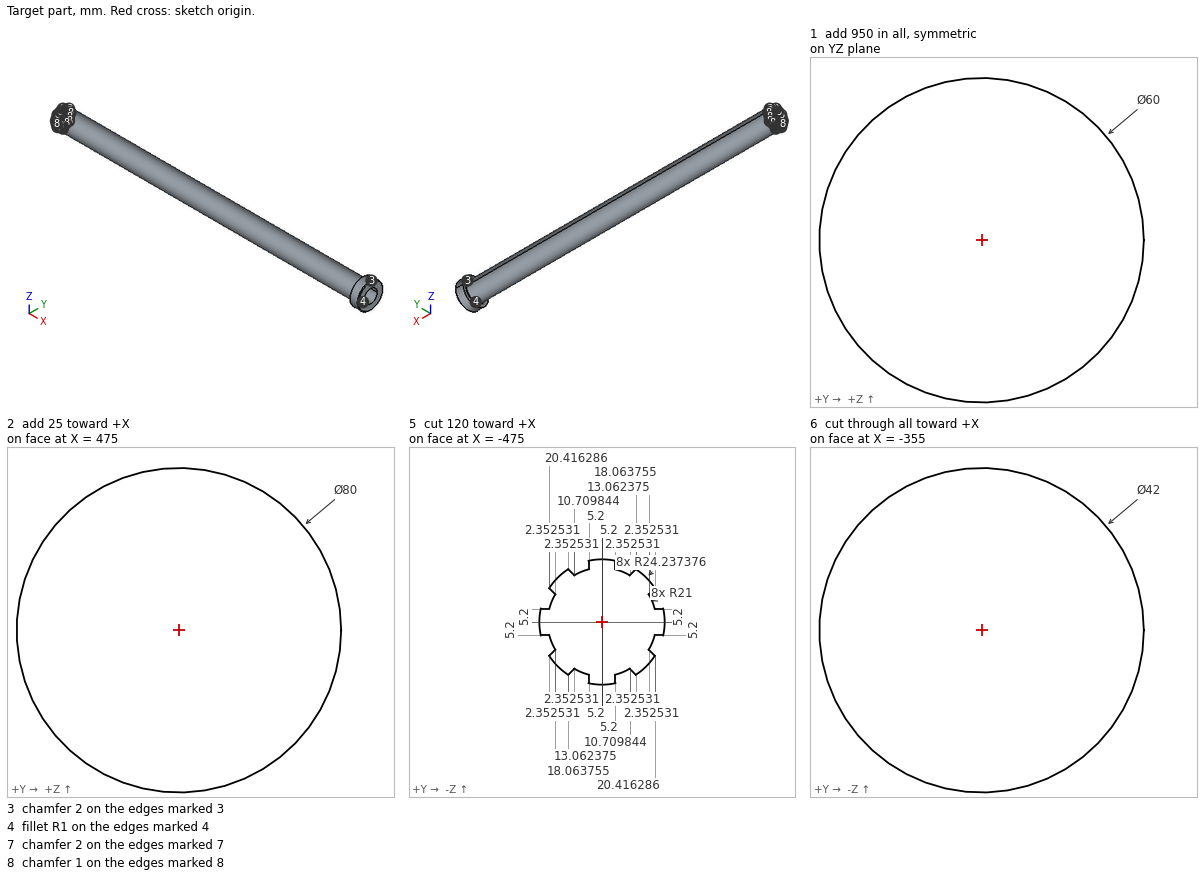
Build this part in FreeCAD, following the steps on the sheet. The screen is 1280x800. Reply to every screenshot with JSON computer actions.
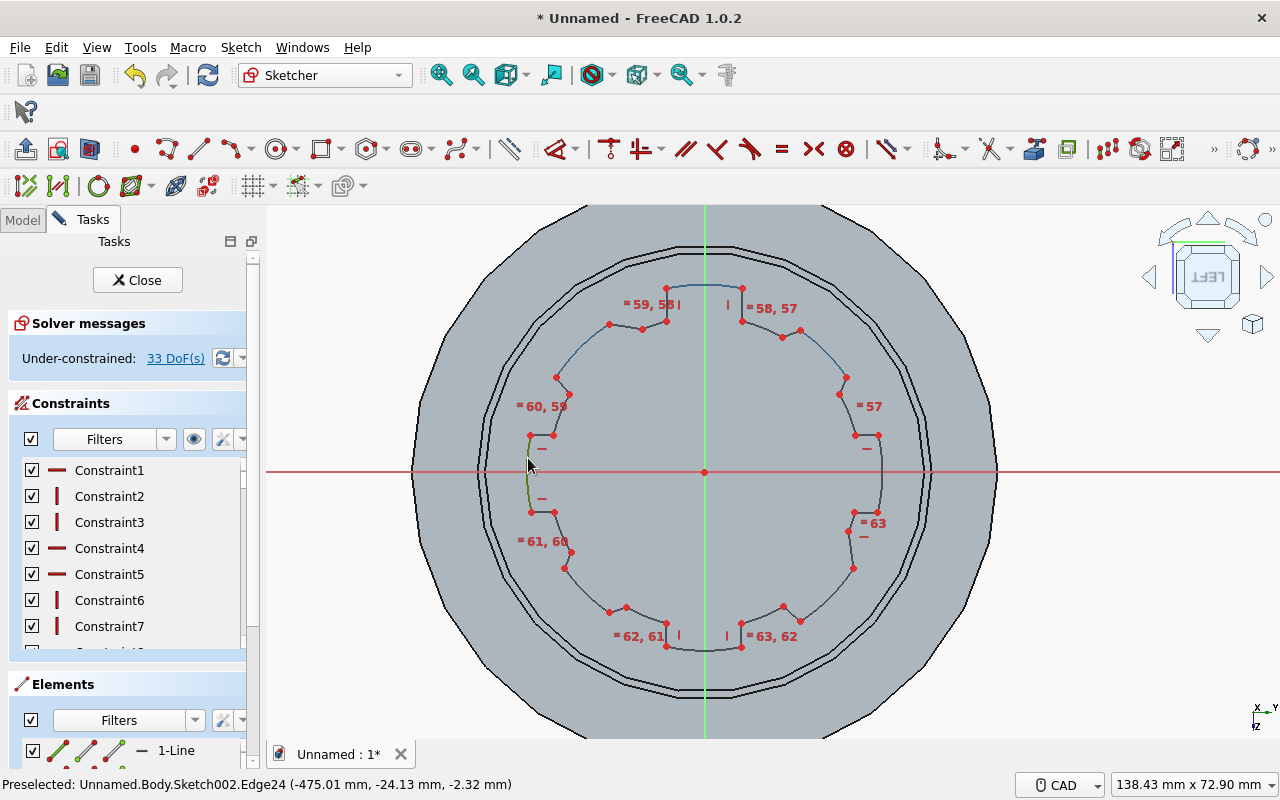
{"action": "left_click", "coordinate": [576, 583]}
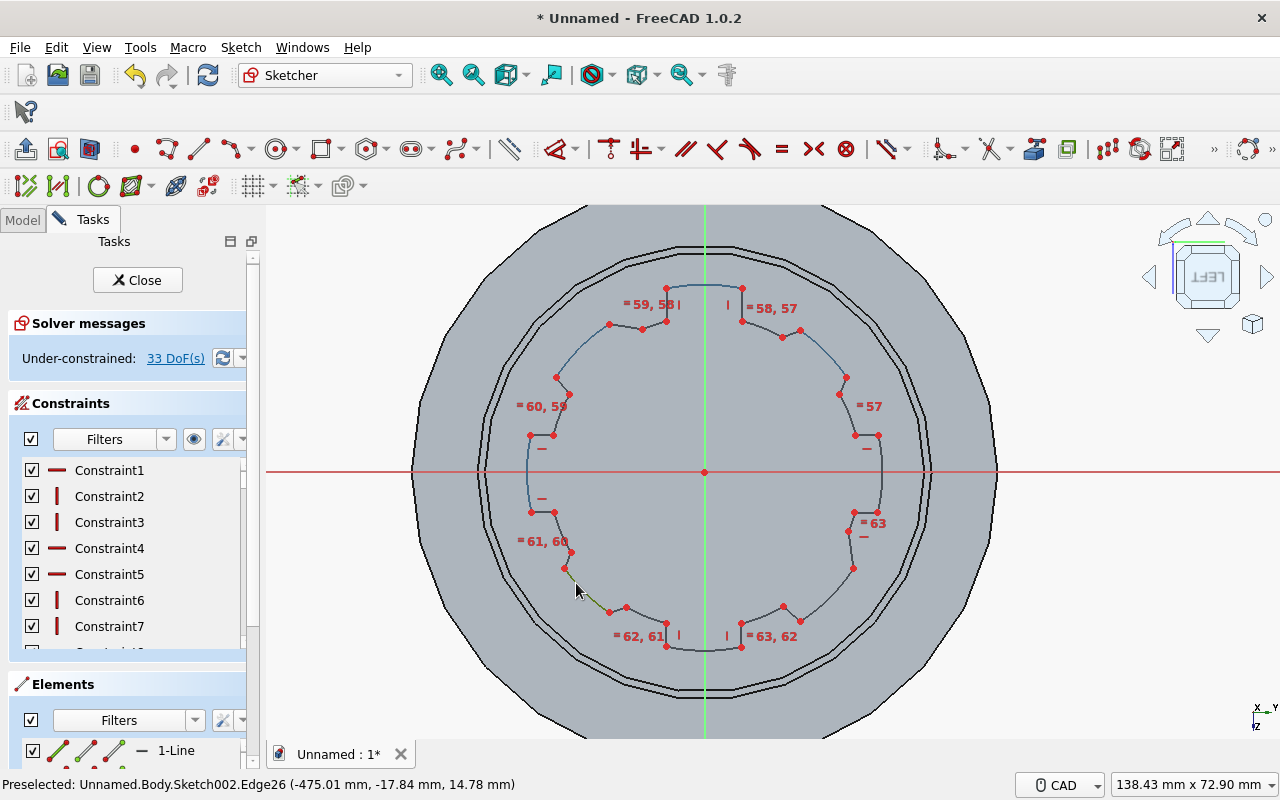
{"action": "left_click", "coordinate": [688, 650]}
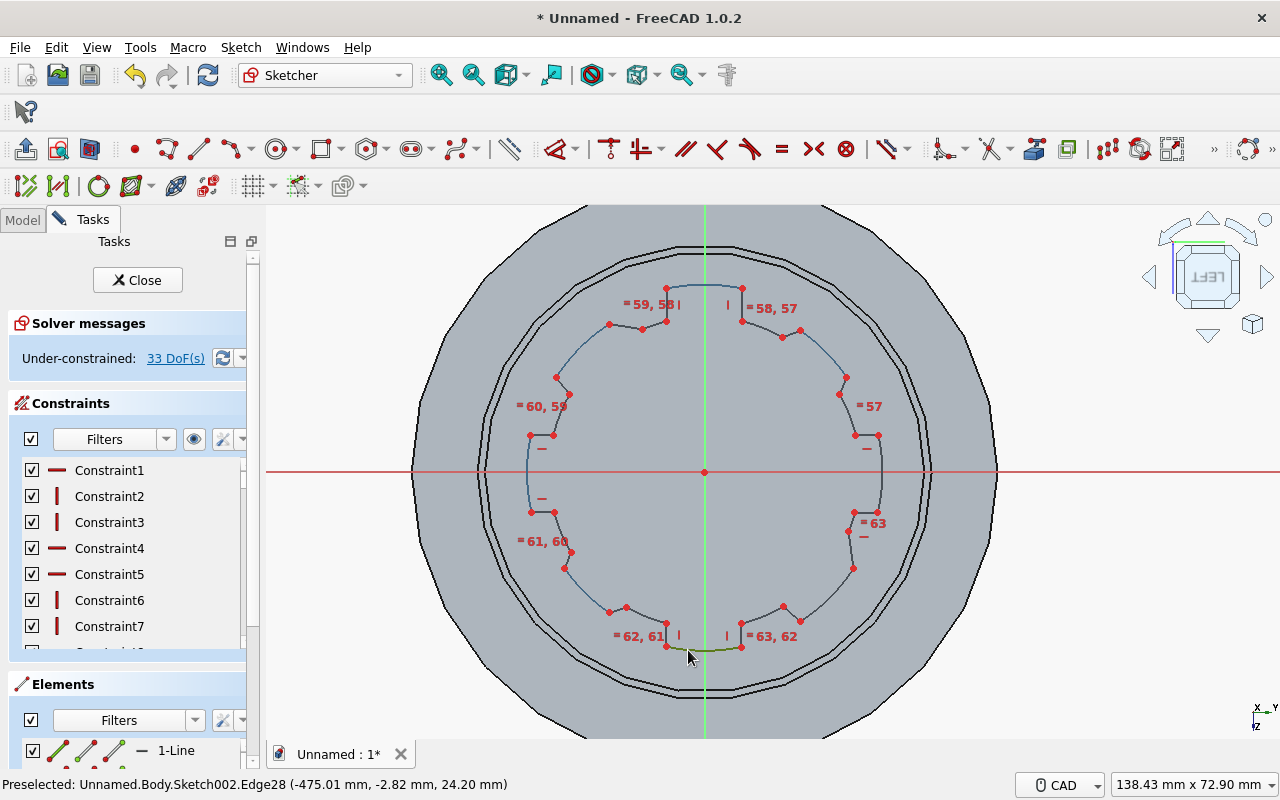
{"action": "left_click", "coordinate": [819, 608]}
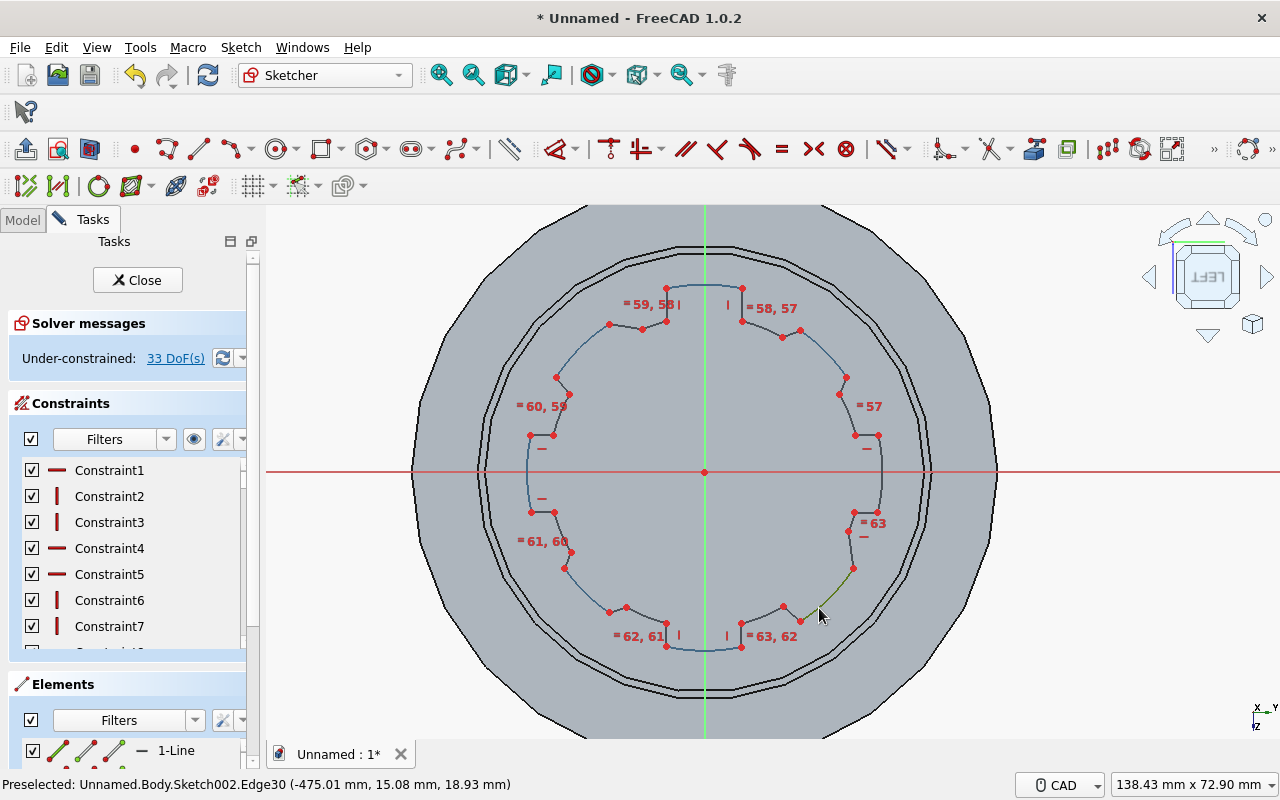
{"action": "left_click", "coordinate": [881, 490]}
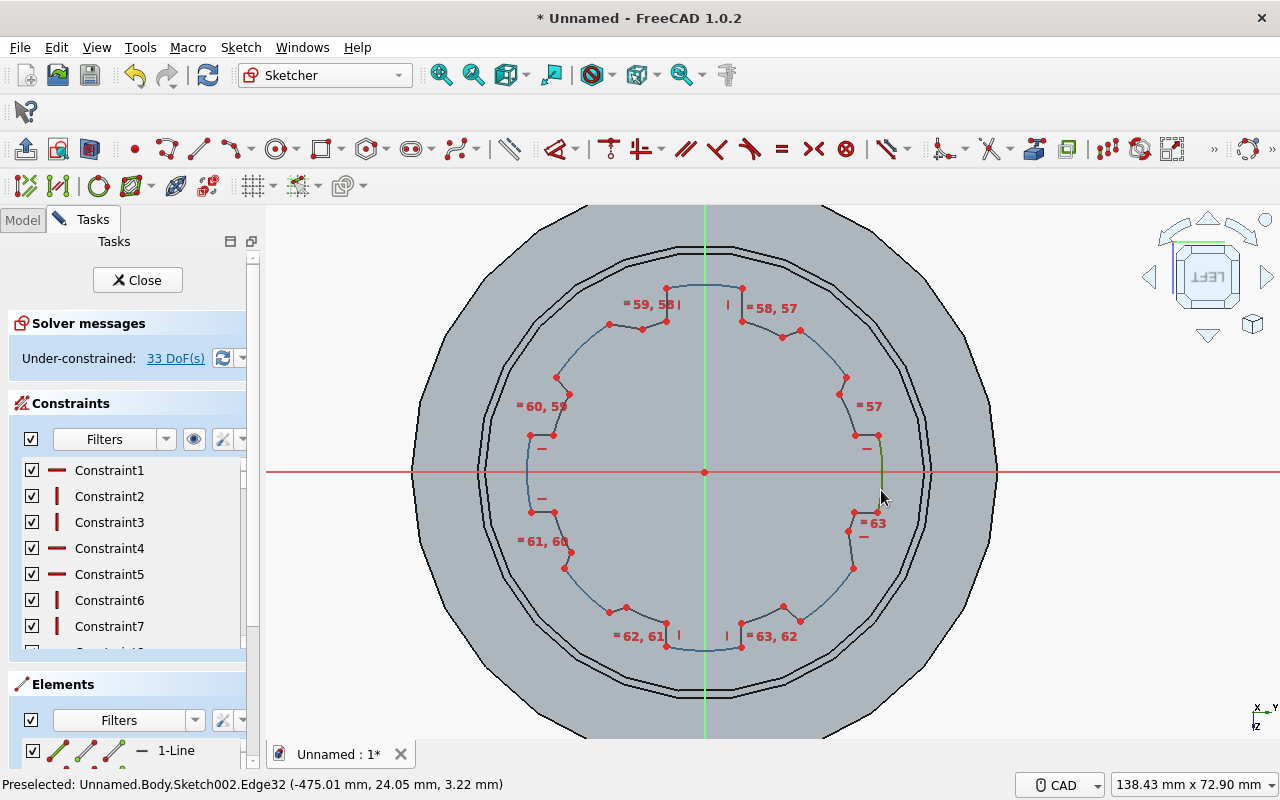
{"action": "key", "text": "e"}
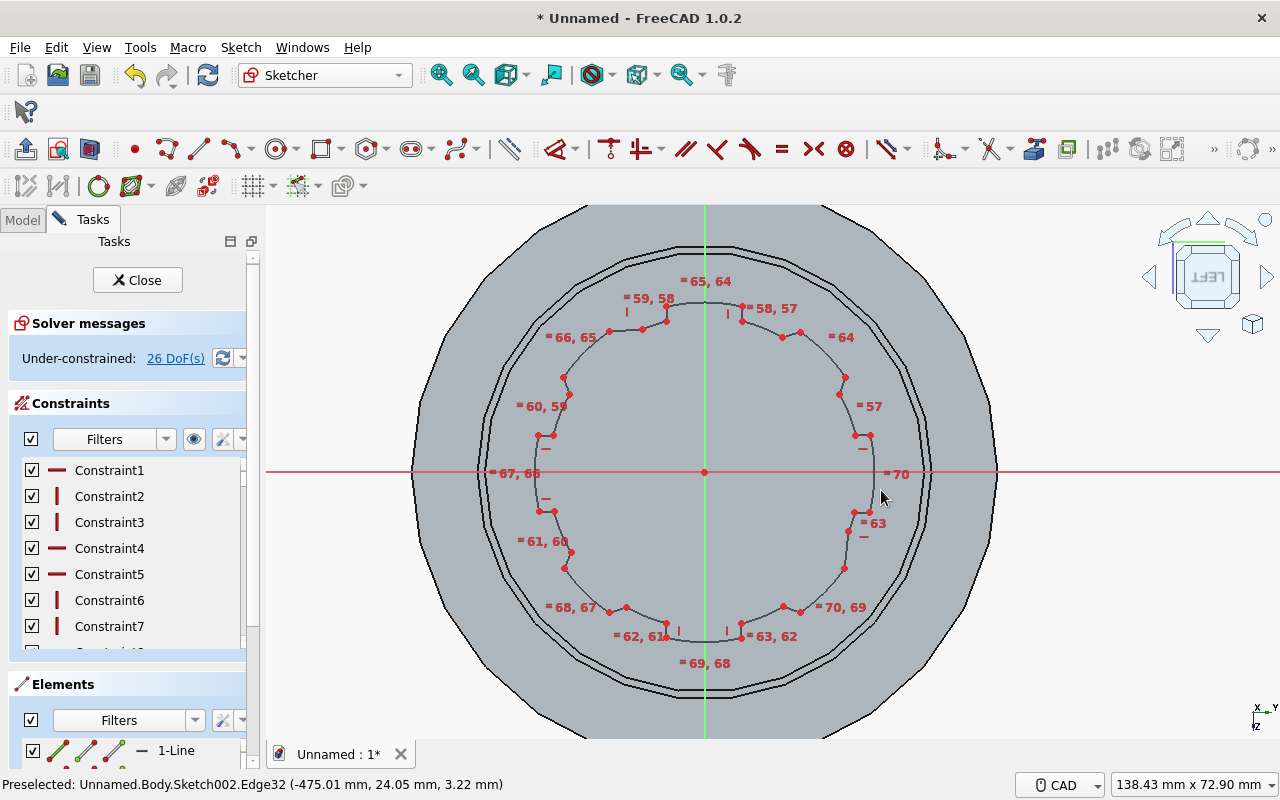
{"action": "key", "text": "d"}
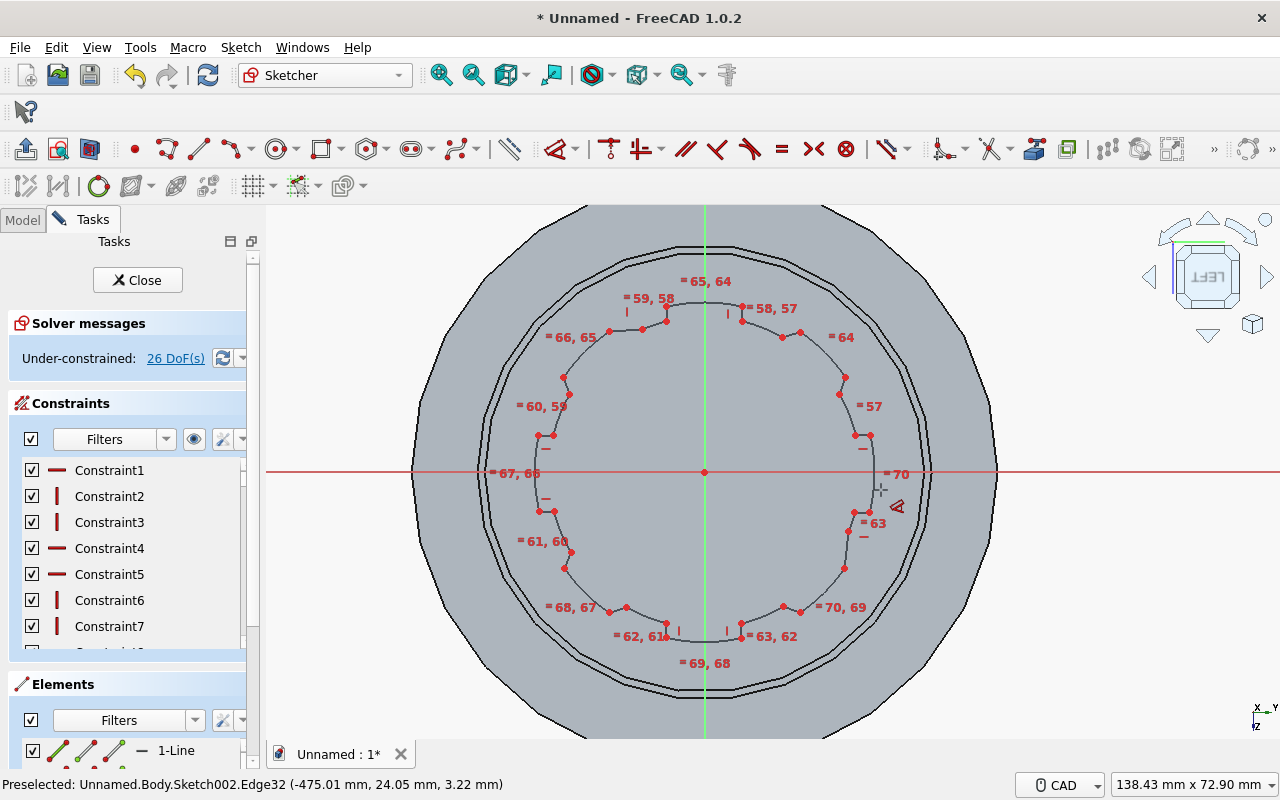
{"action": "left_click", "coordinate": [852, 423]}
{"action": "left_click", "coordinate": [882, 413]}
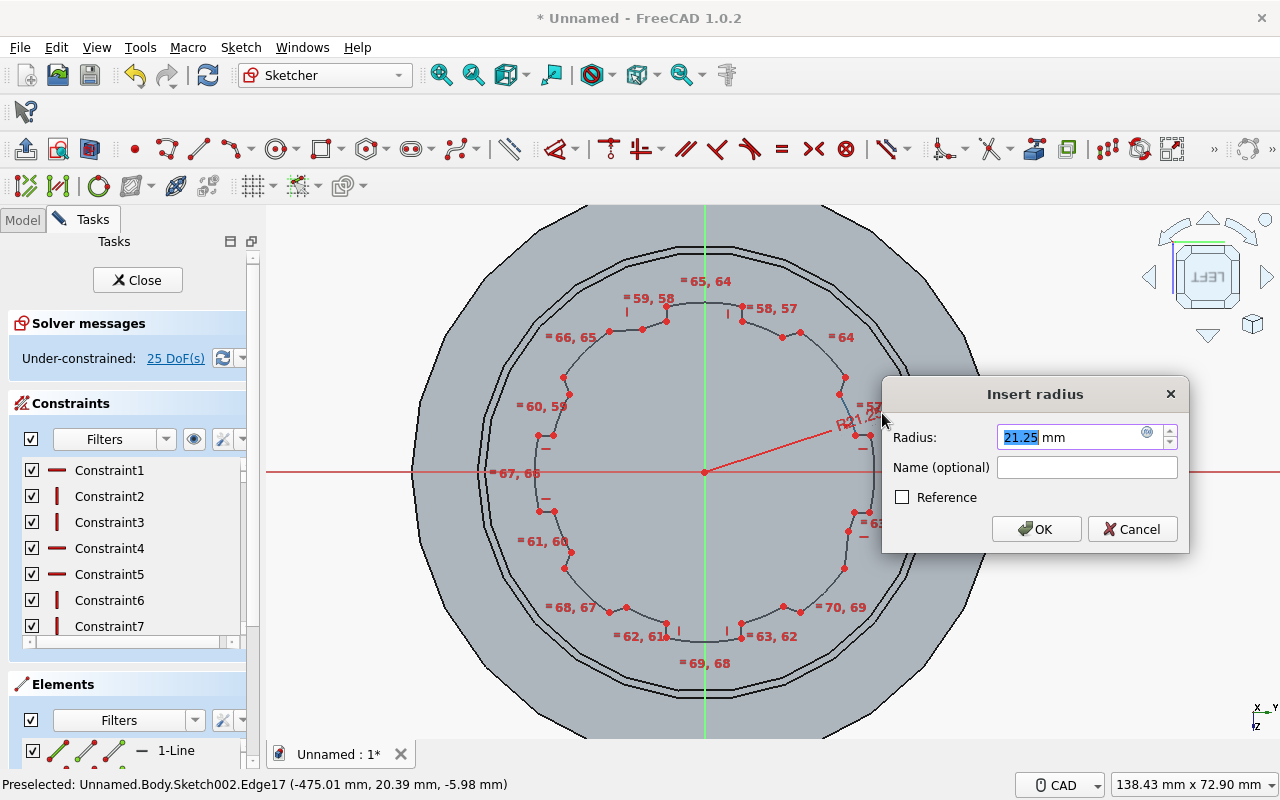
{"action": "type", "text": "21"}
{"action": "key", "text": "Return"}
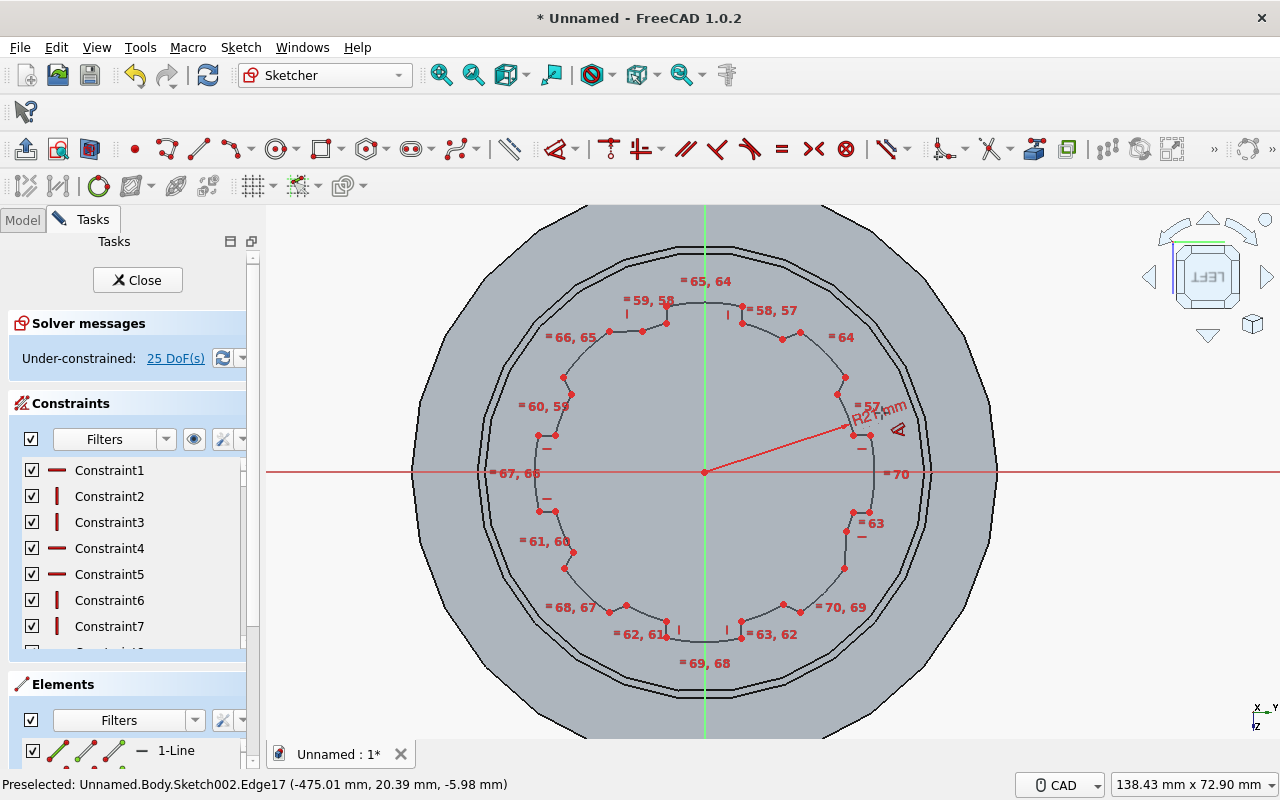
{"action": "left_click", "coordinate": [834, 362]}
{"action": "left_click", "coordinate": [858, 341]}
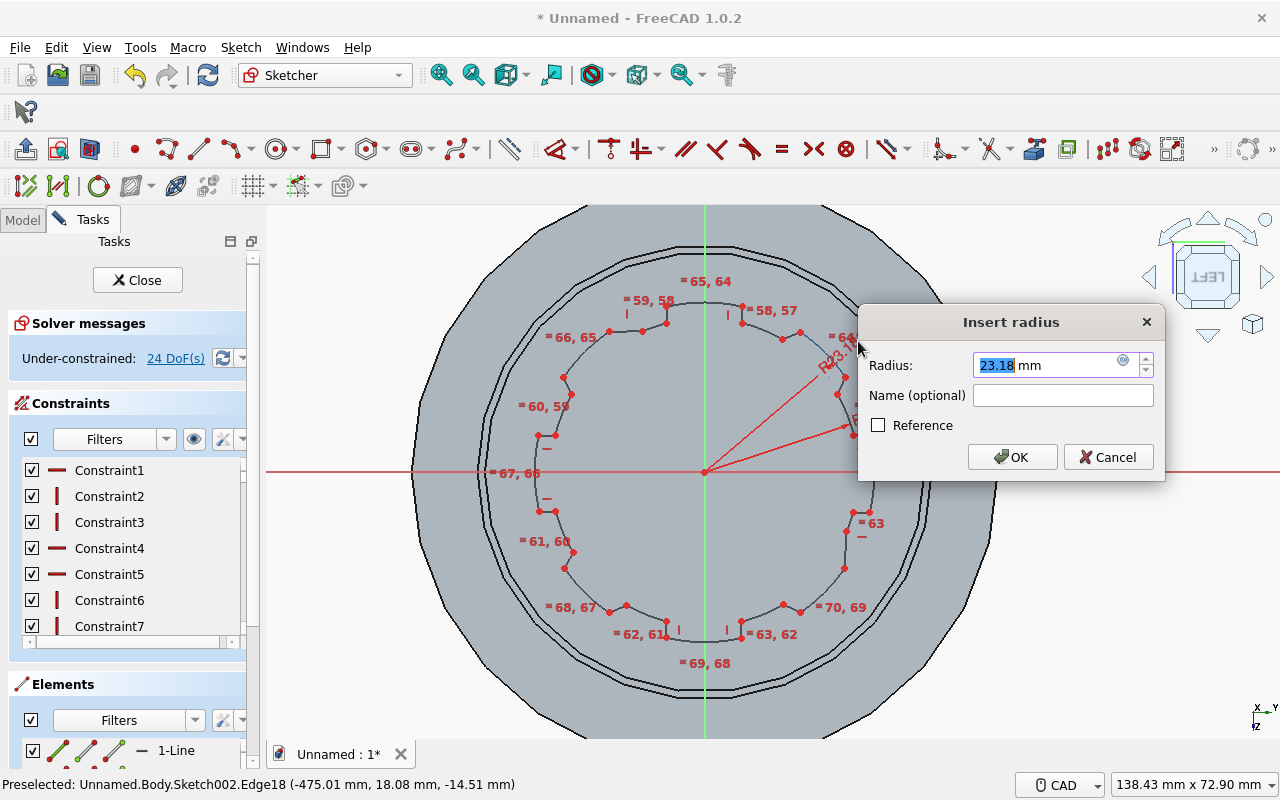
{"action": "type", "text": "24.237376"}
{"action": "key", "text": "Return"}